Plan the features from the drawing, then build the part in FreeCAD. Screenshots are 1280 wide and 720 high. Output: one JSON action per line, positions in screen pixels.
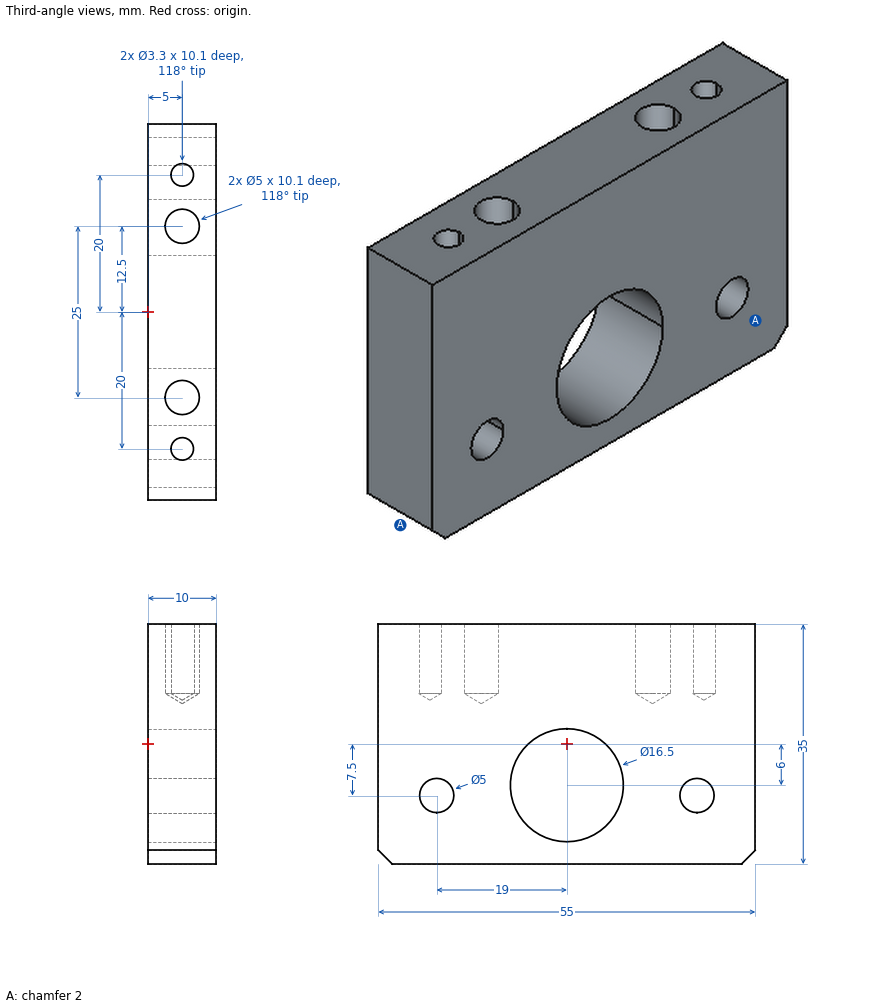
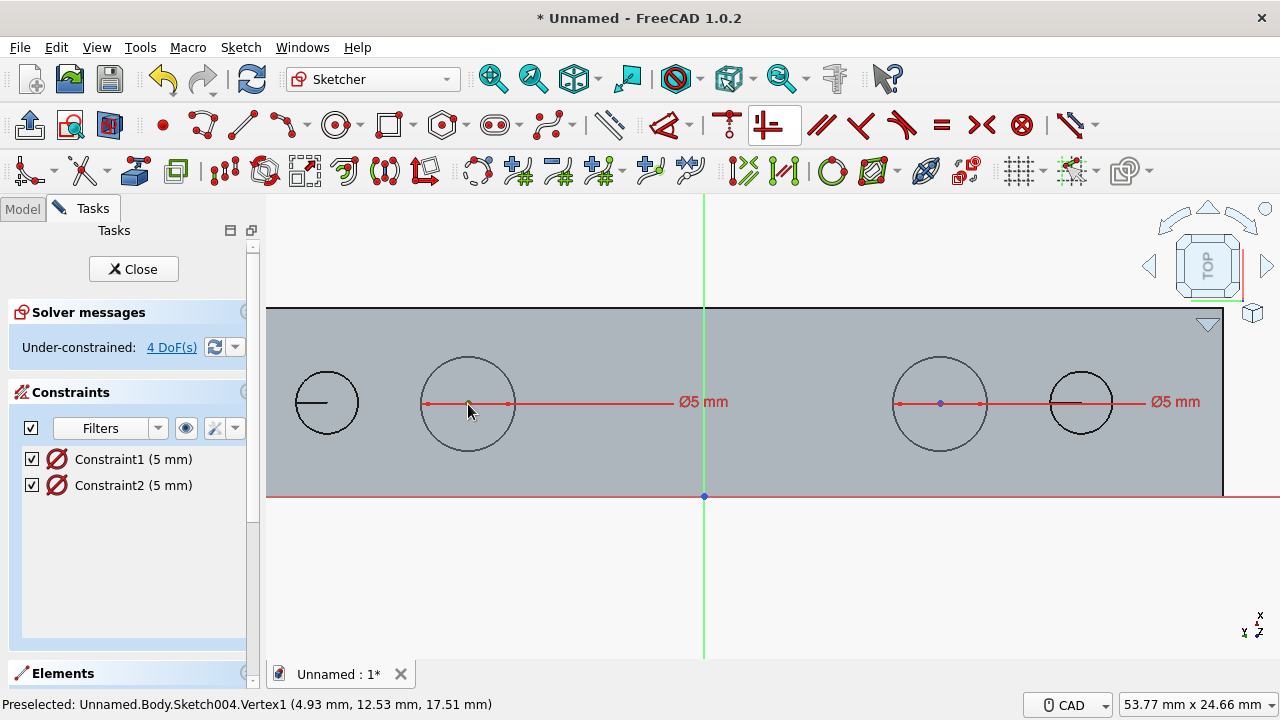
{"action": "left_click", "coordinate": [940, 404]}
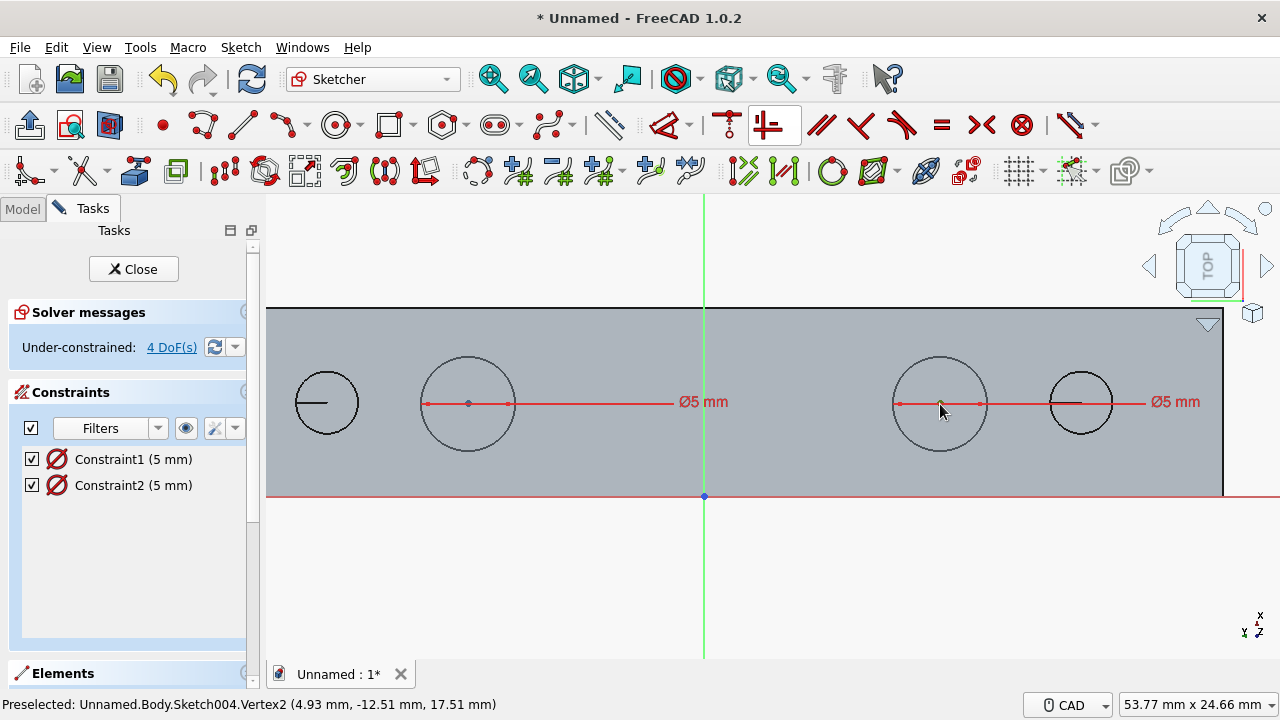
{"action": "left_click", "coordinate": [796, 126]}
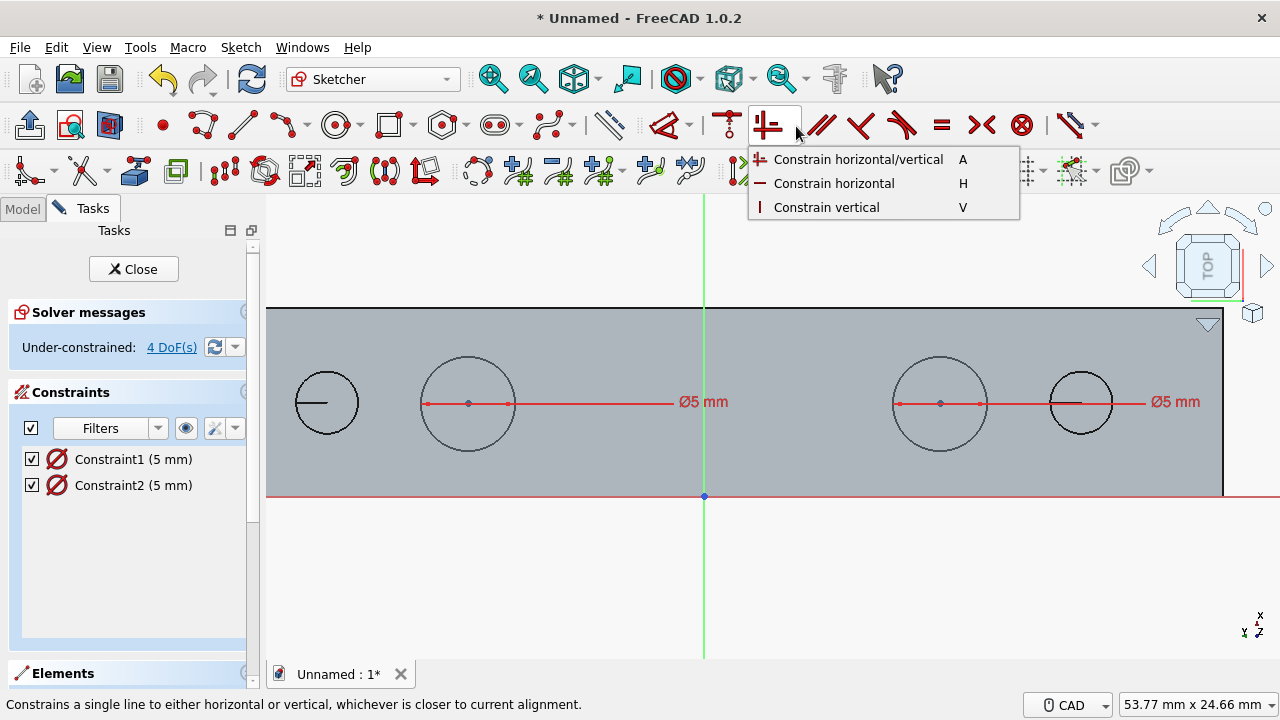
{"action": "left_click", "coordinate": [884, 183]}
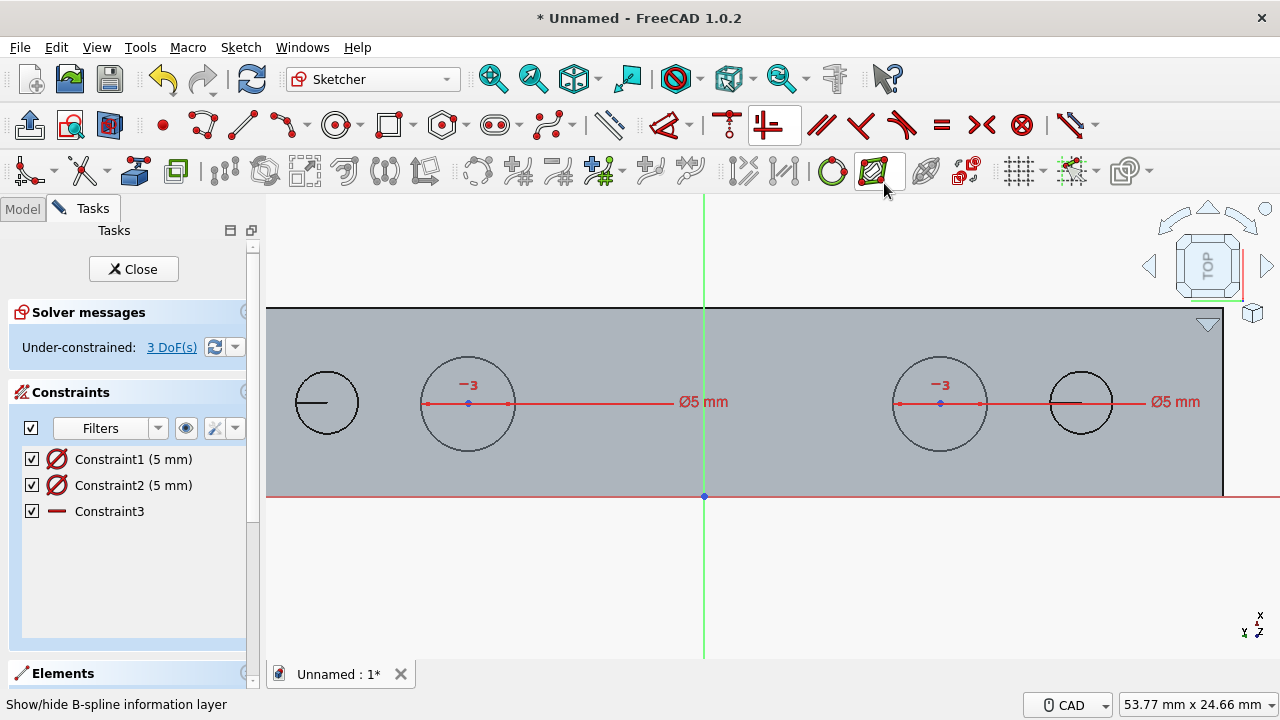
{"action": "left_click", "coordinate": [664, 126]}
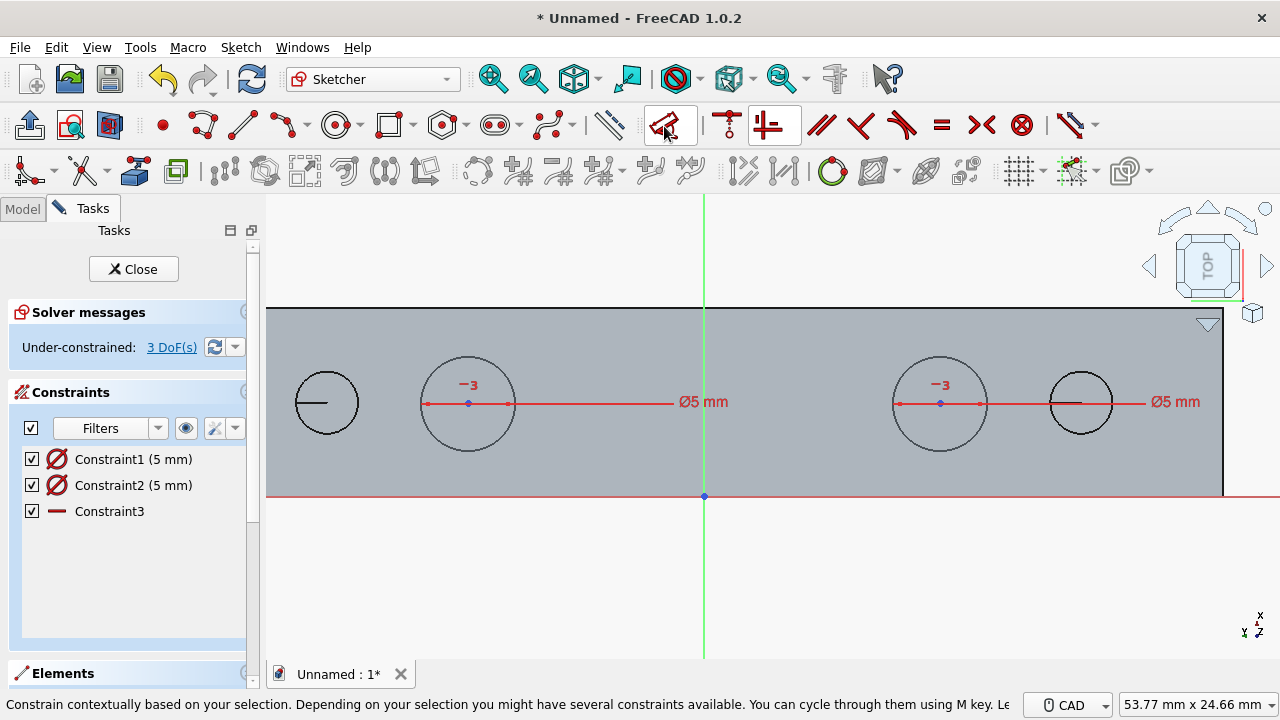
{"action": "left_click", "coordinate": [468, 404]}
{"action": "left_click", "coordinate": [434, 472]}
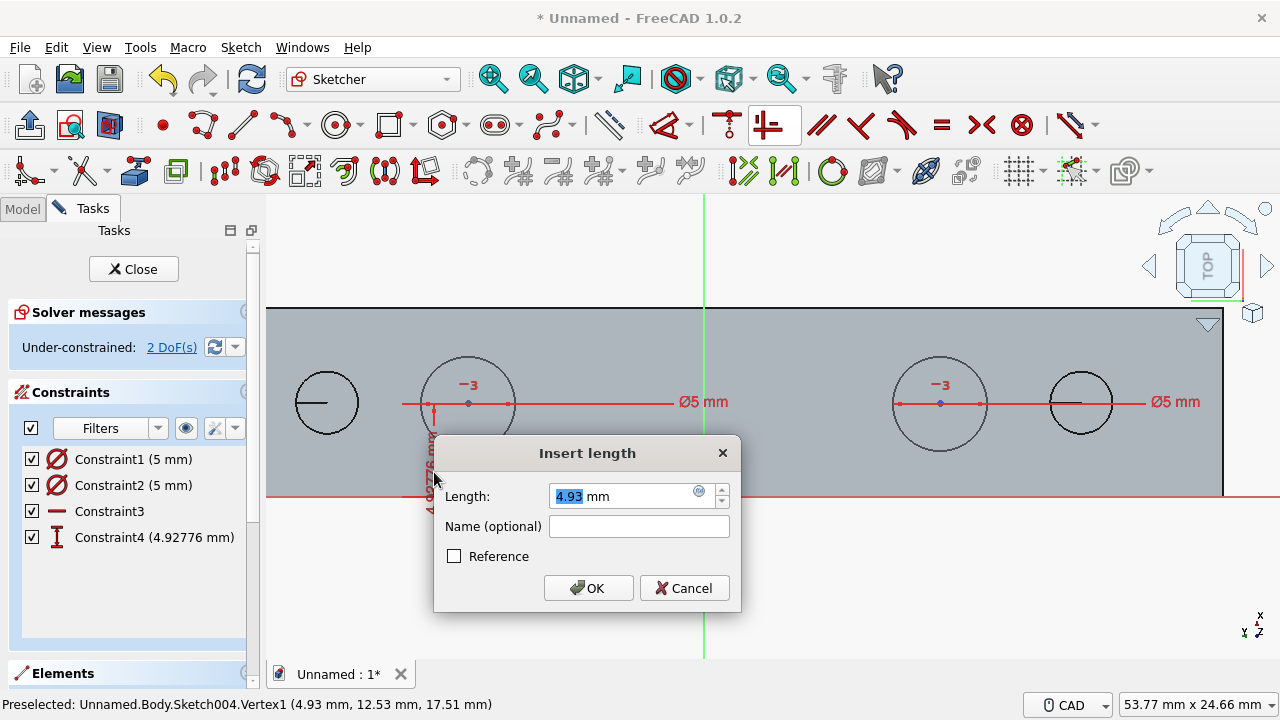
{"action": "type", "text": "5"}
{"action": "key", "text": "Return"}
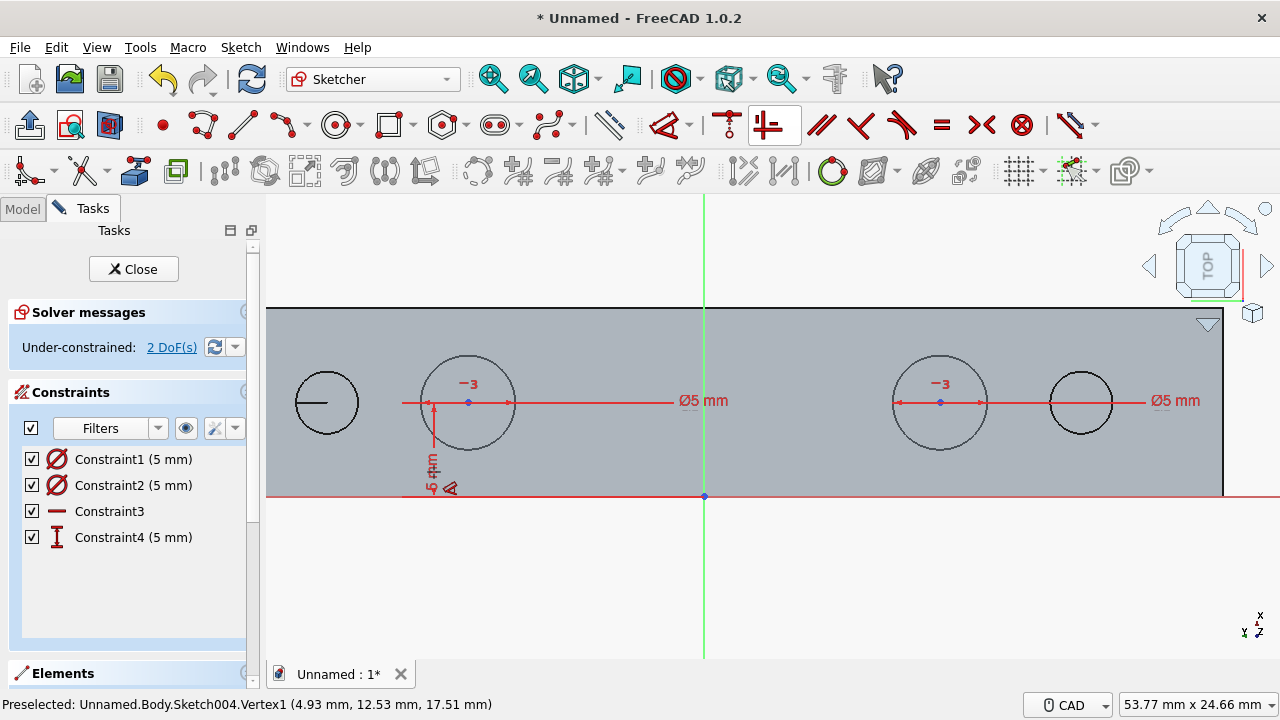
{"action": "left_click", "coordinate": [468, 403]}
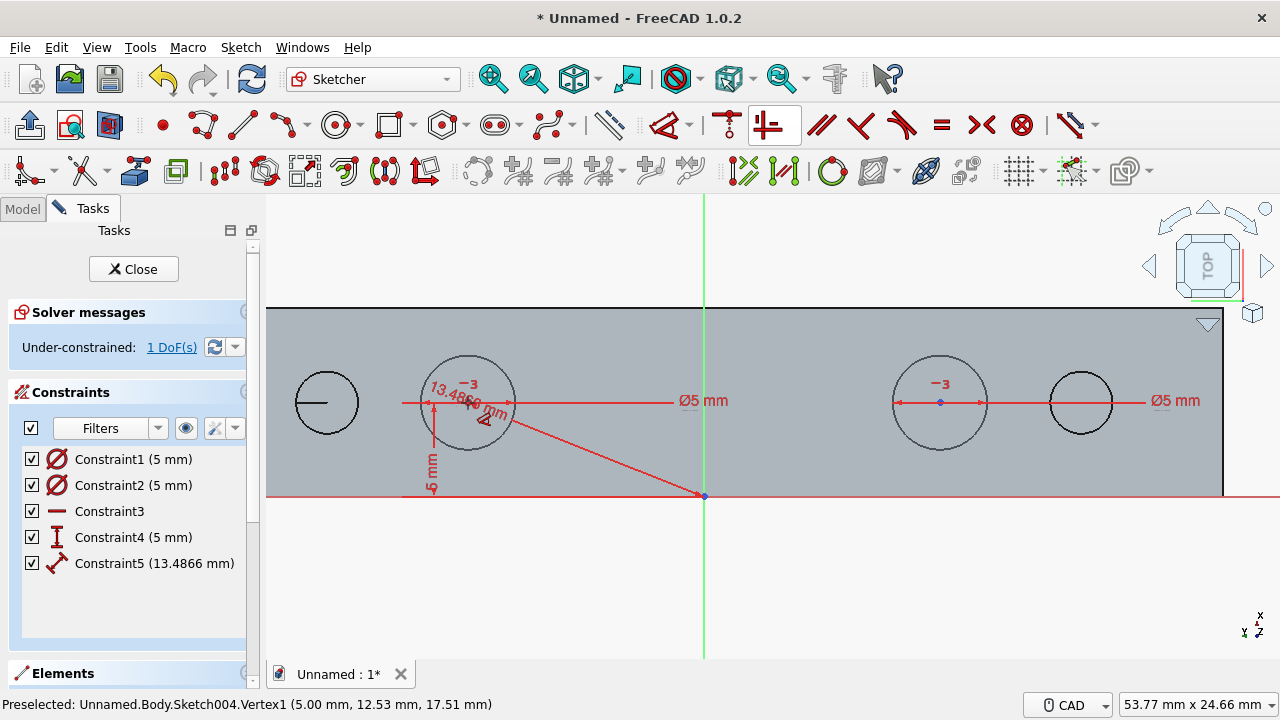
{"action": "left_click", "coordinate": [940, 403]}
{"action": "left_click", "coordinate": [595, 369]}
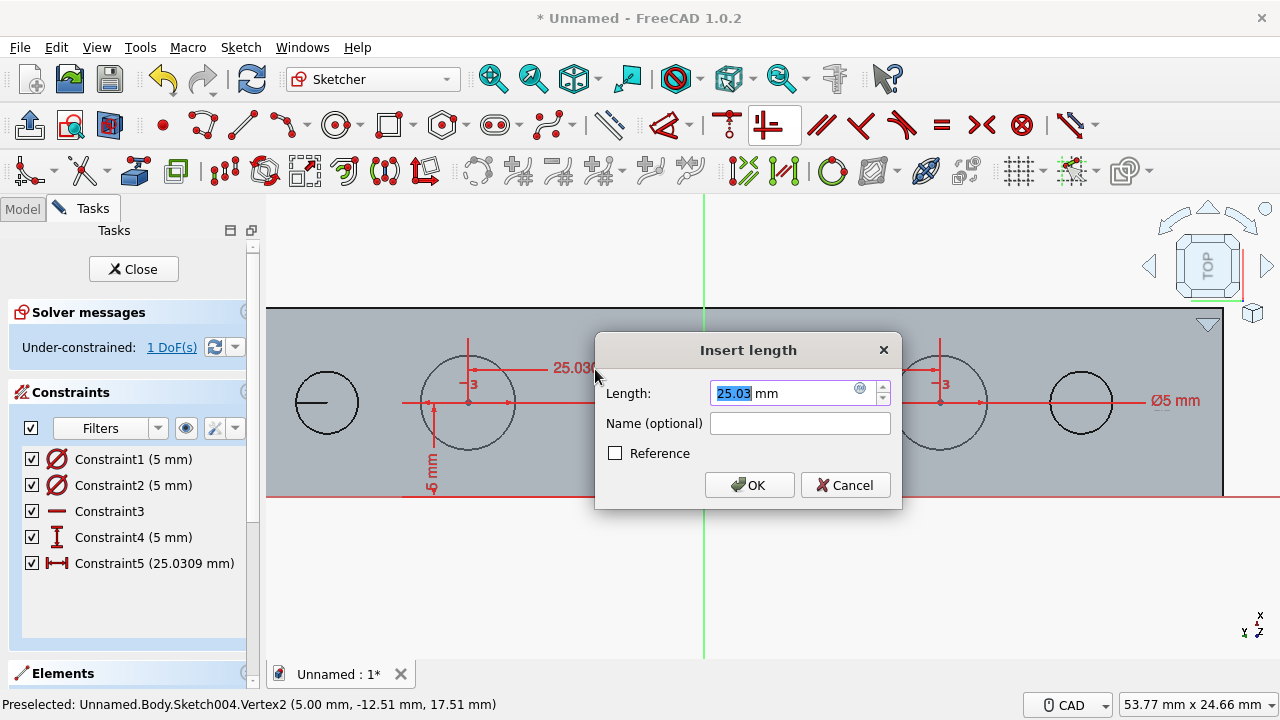
{"action": "type", "text": "25"}
{"action": "key", "text": "Return"}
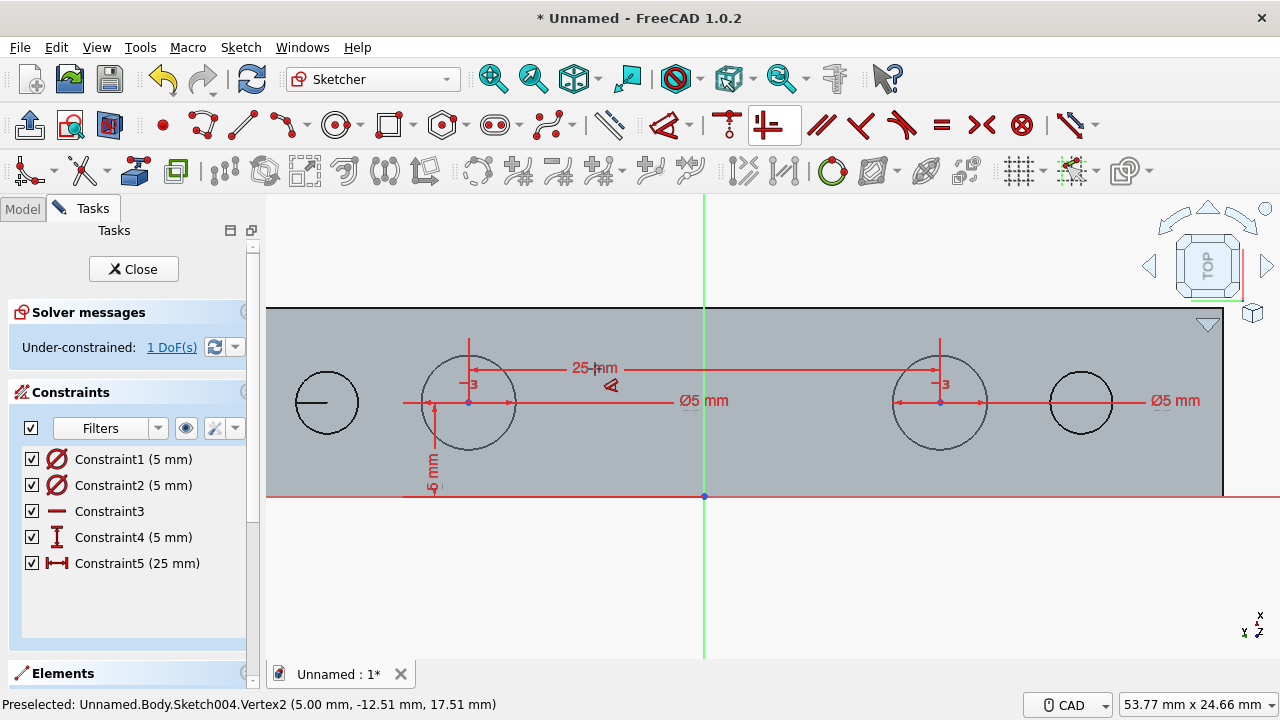
{"action": "left_click", "coordinate": [469, 403]}
{"action": "left_click", "coordinate": [586, 531]}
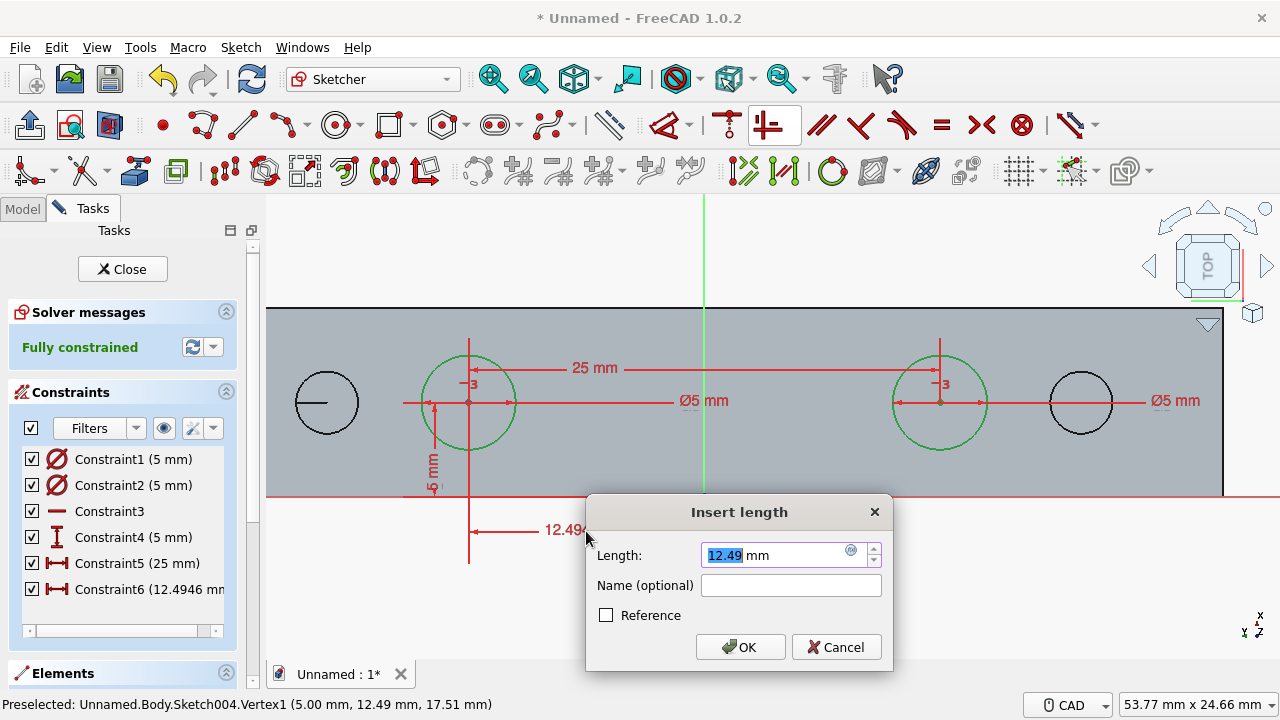
{"action": "type", "text": "12.5"}
{"action": "key", "text": "Return"}
{"action": "key", "text": "Escape"}